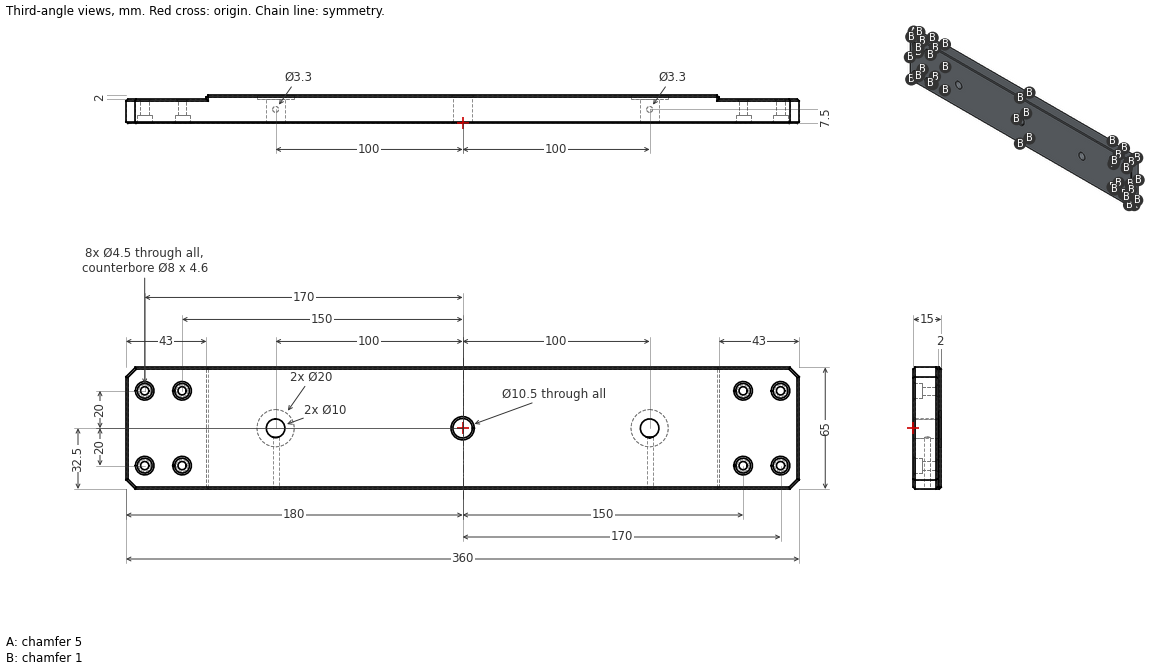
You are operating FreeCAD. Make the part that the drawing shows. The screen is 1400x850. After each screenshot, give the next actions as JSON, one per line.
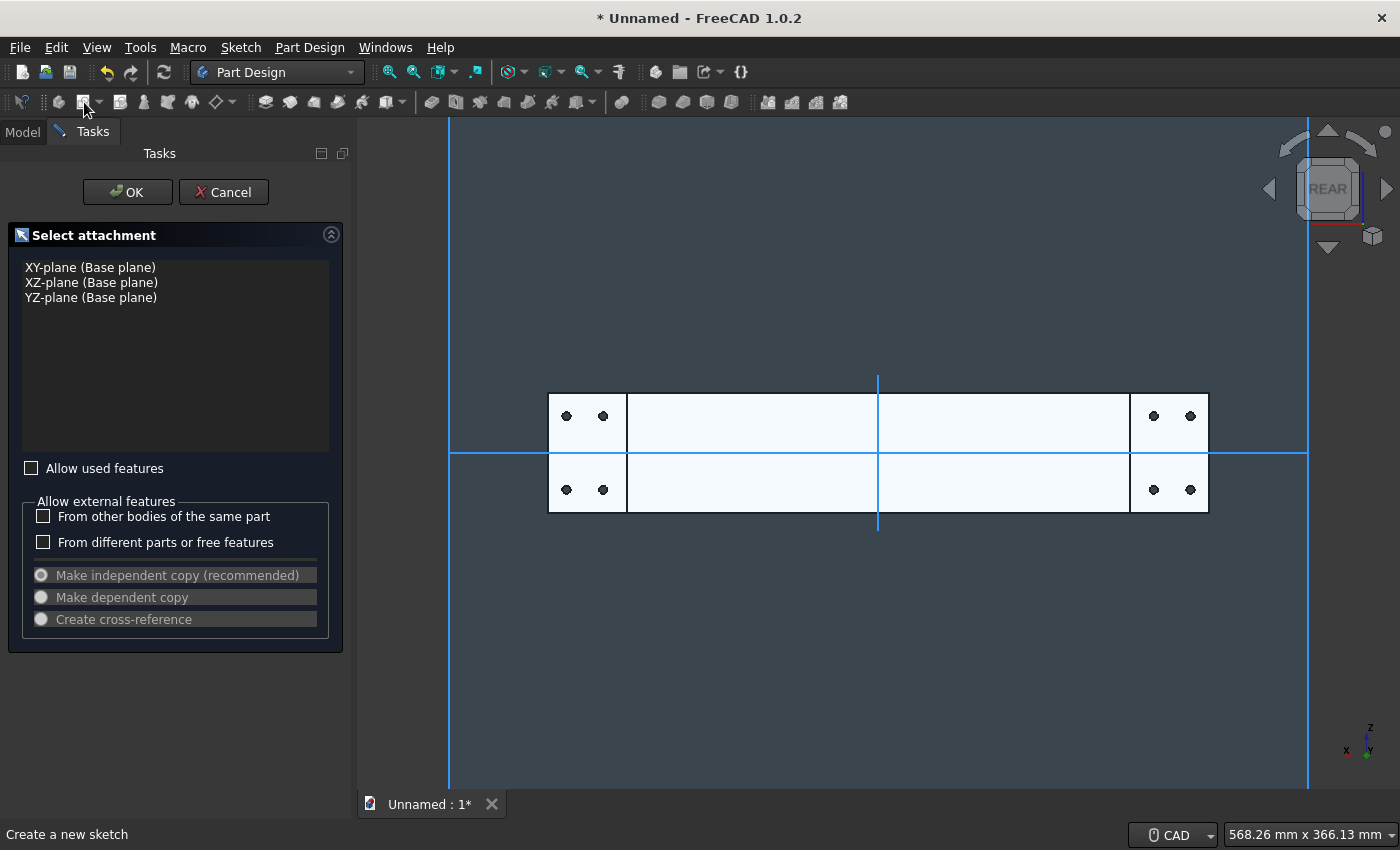
{"action": "left_click", "coordinate": [82, 282]}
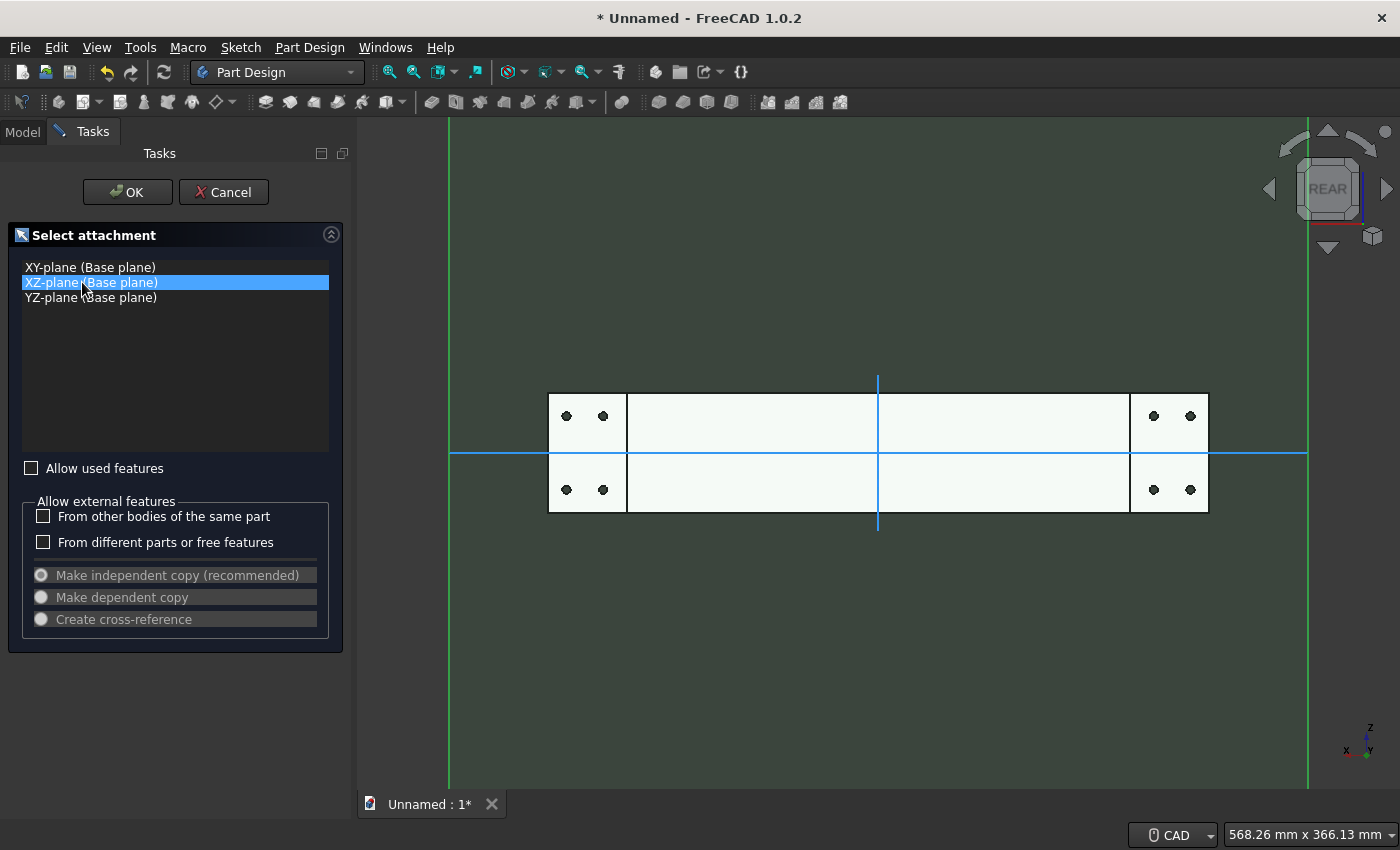
{"action": "left_click", "coordinate": [128, 192]}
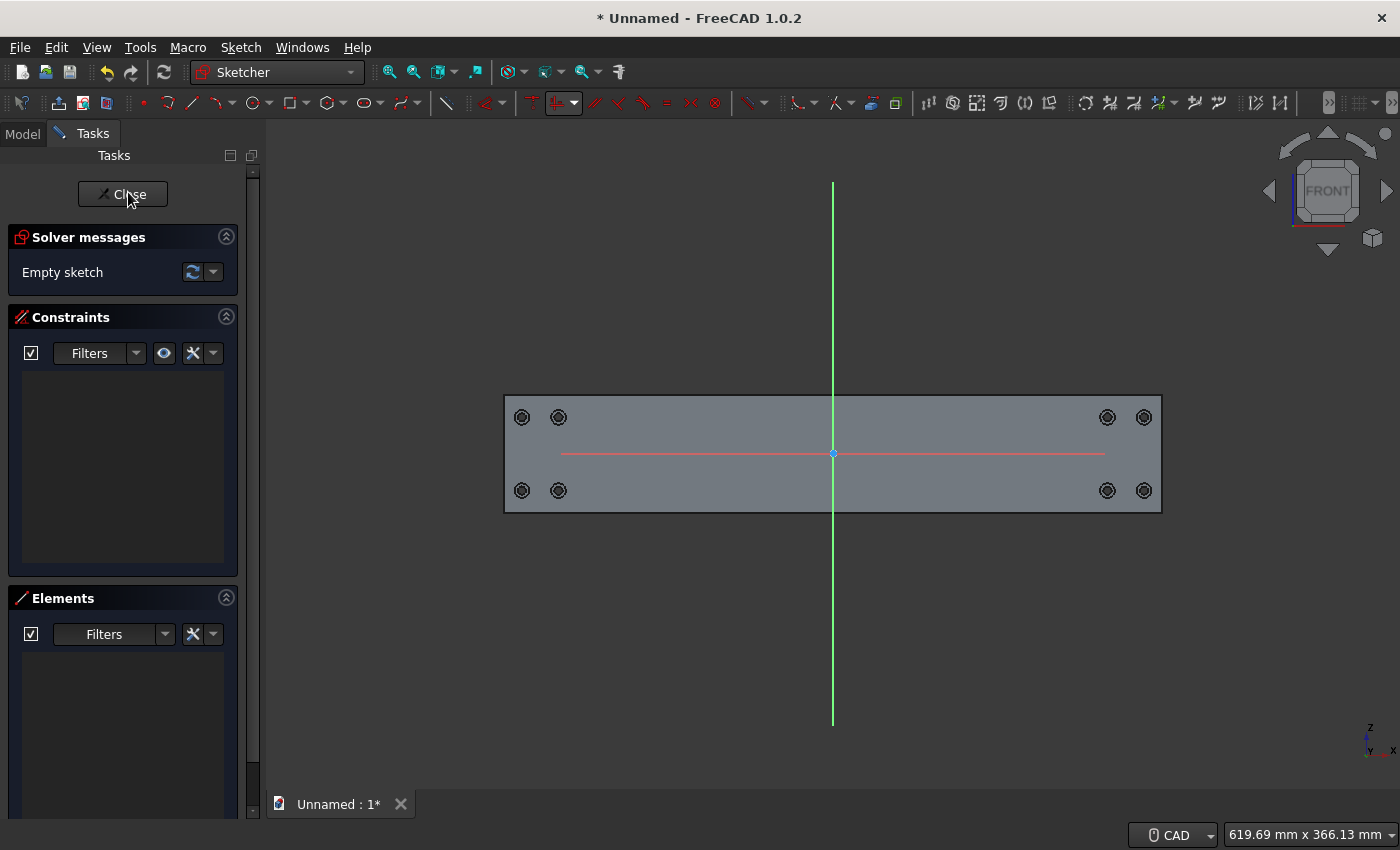
{"action": "scroll", "coordinate": [837, 454], "scroll_direction": "up", "scroll_amount": 15}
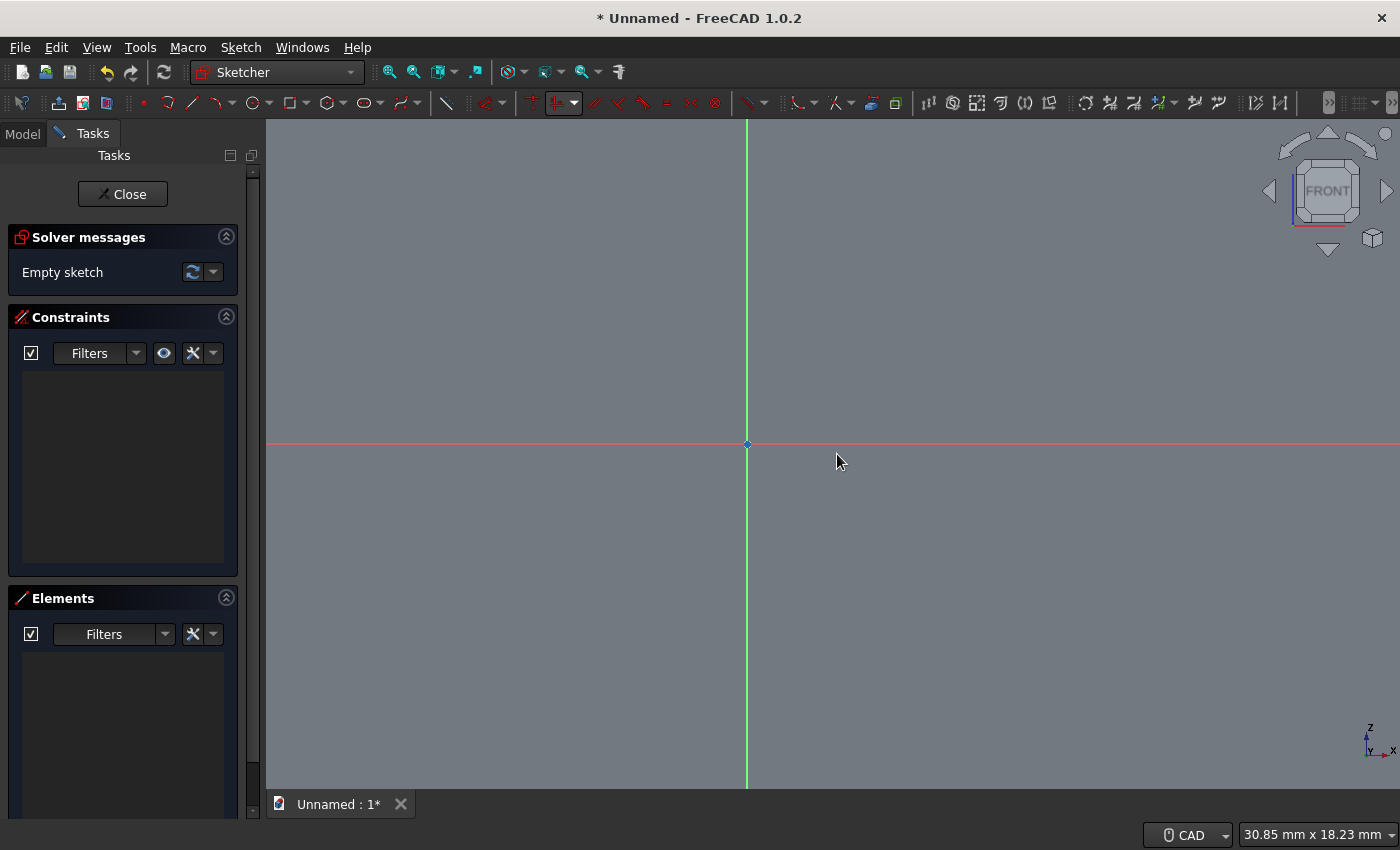
{"action": "left_click", "coordinate": [254, 104]}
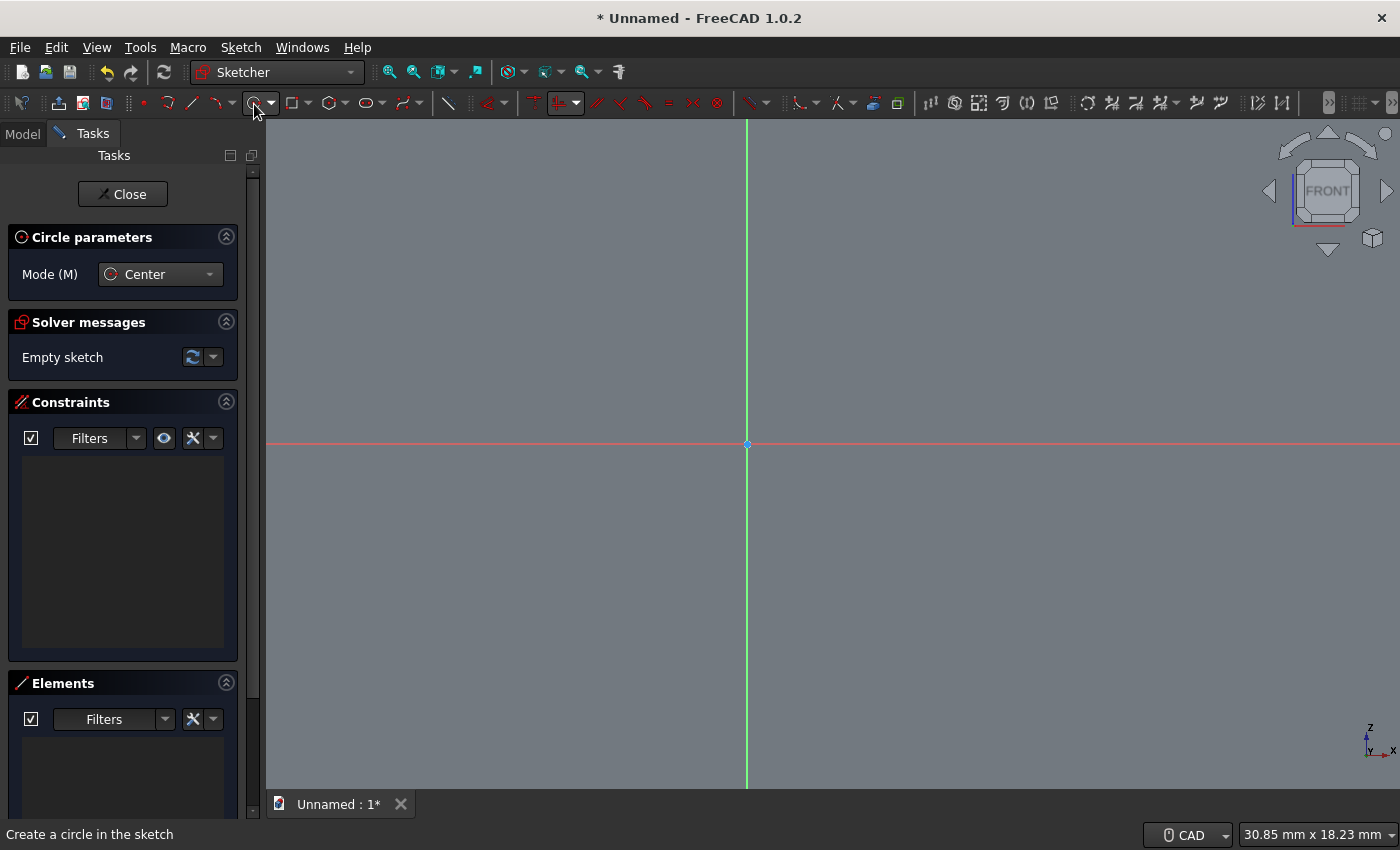
{"action": "left_click", "coordinate": [747, 444]}
{"action": "mouse_move", "coordinate": [883, 308]}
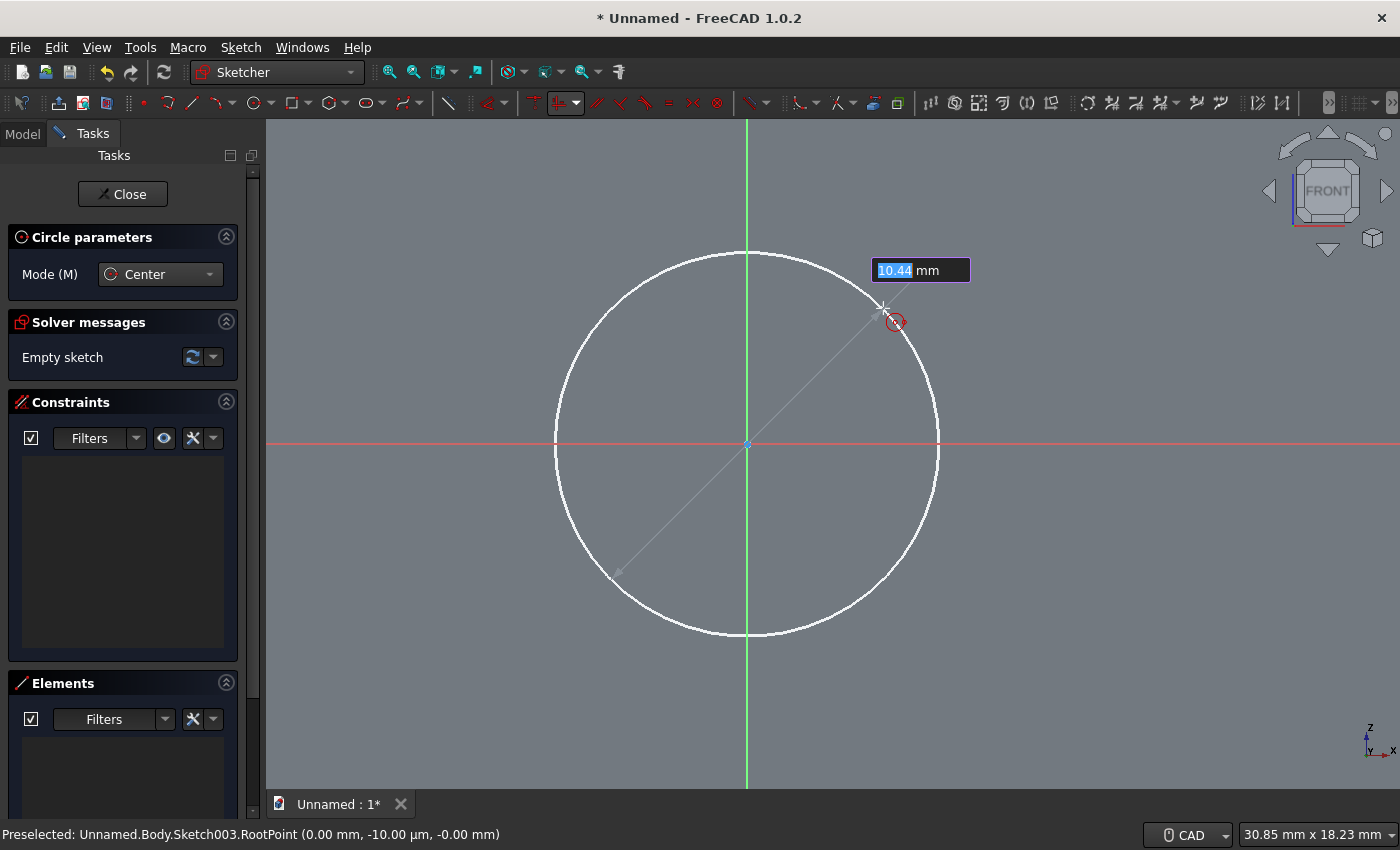
{"action": "type", "text": "10.5"}
{"action": "key", "text": "Return"}
{"action": "key", "text": "Escape"}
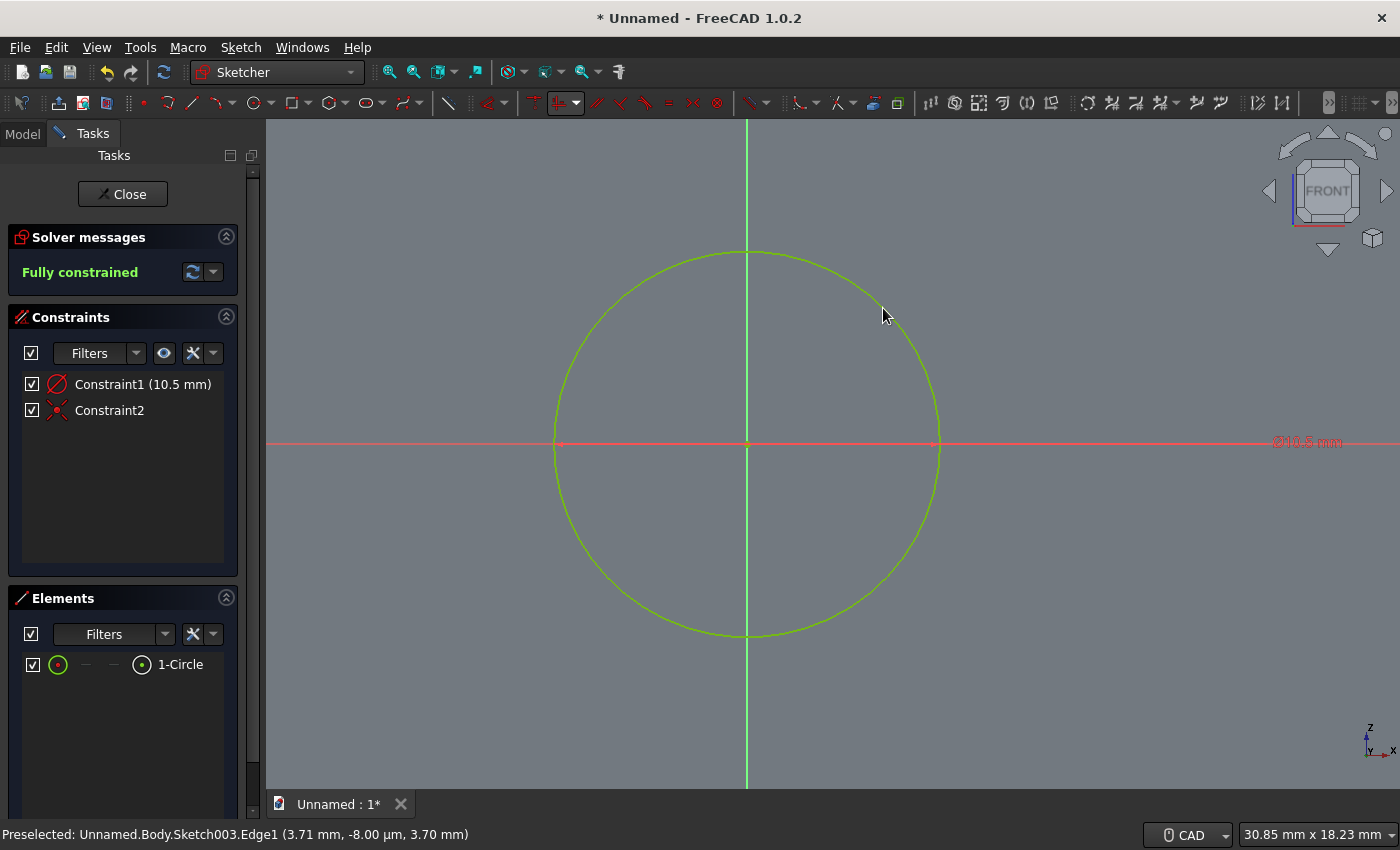
{"action": "left_click", "coordinate": [123, 194]}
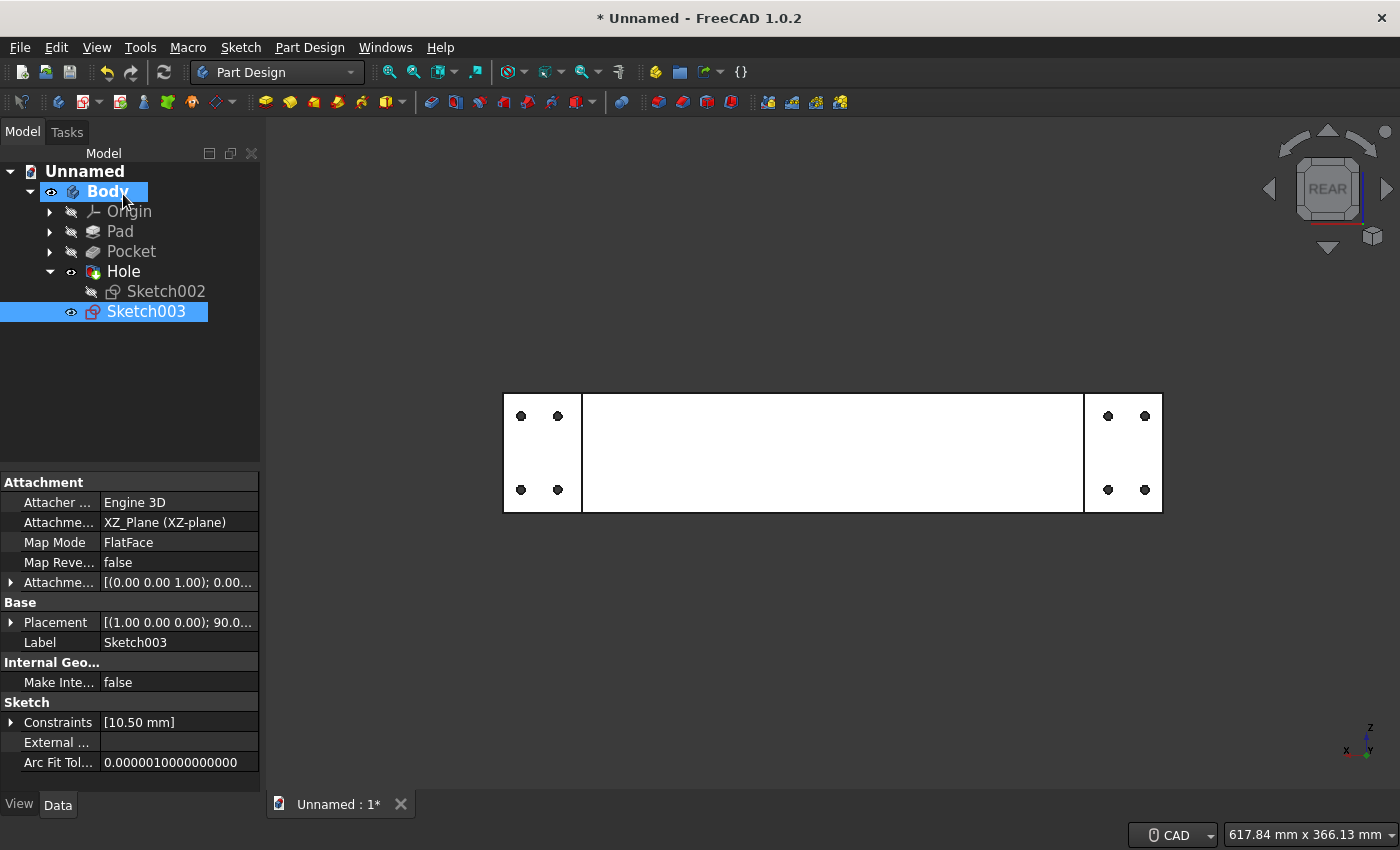
{"action": "left_click", "coordinate": [456, 102]}